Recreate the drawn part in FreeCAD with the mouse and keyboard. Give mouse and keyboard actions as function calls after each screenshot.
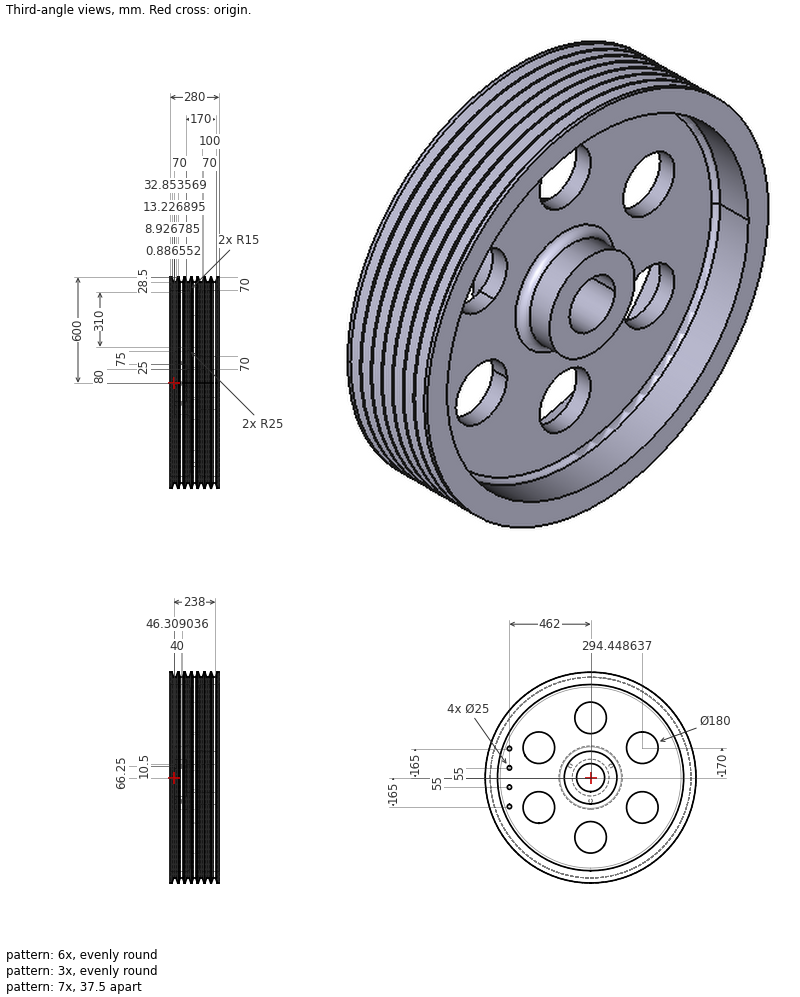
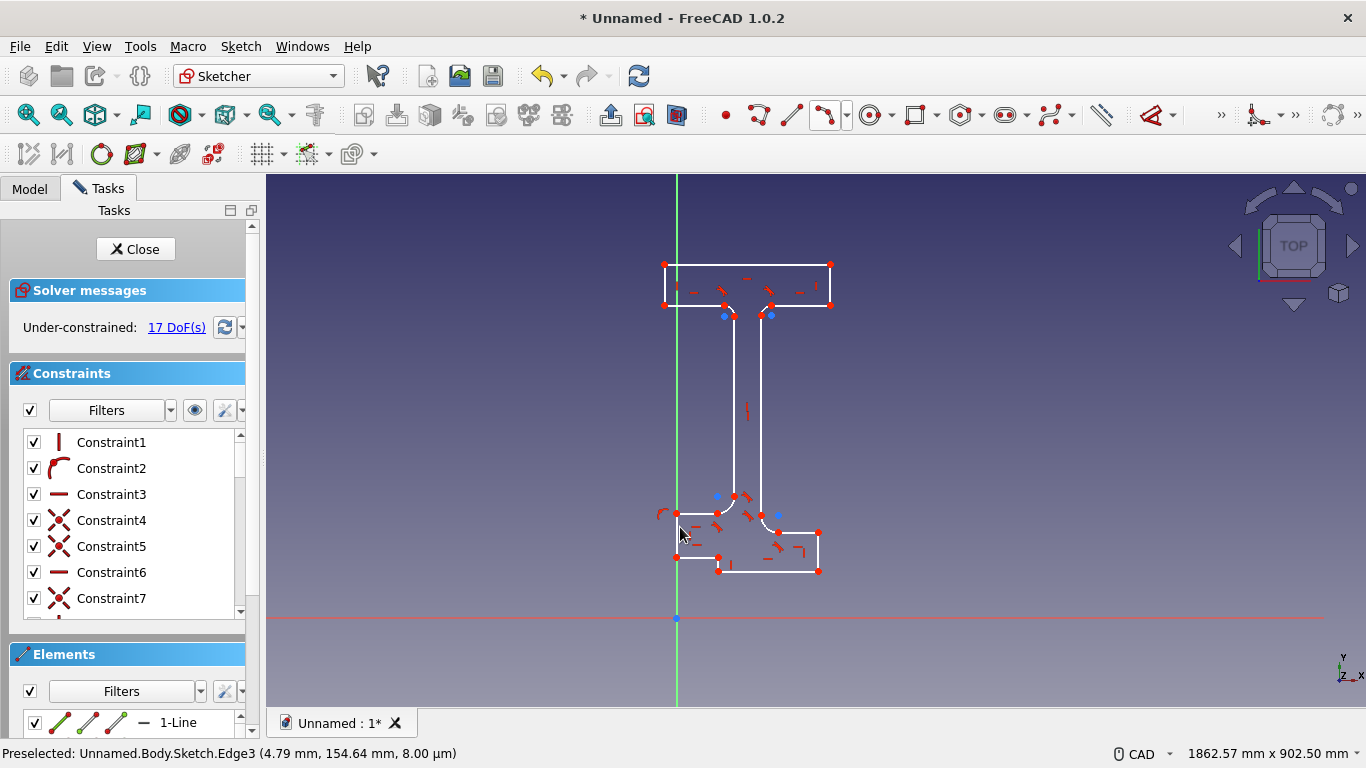
scroll(725, 512, up, 3)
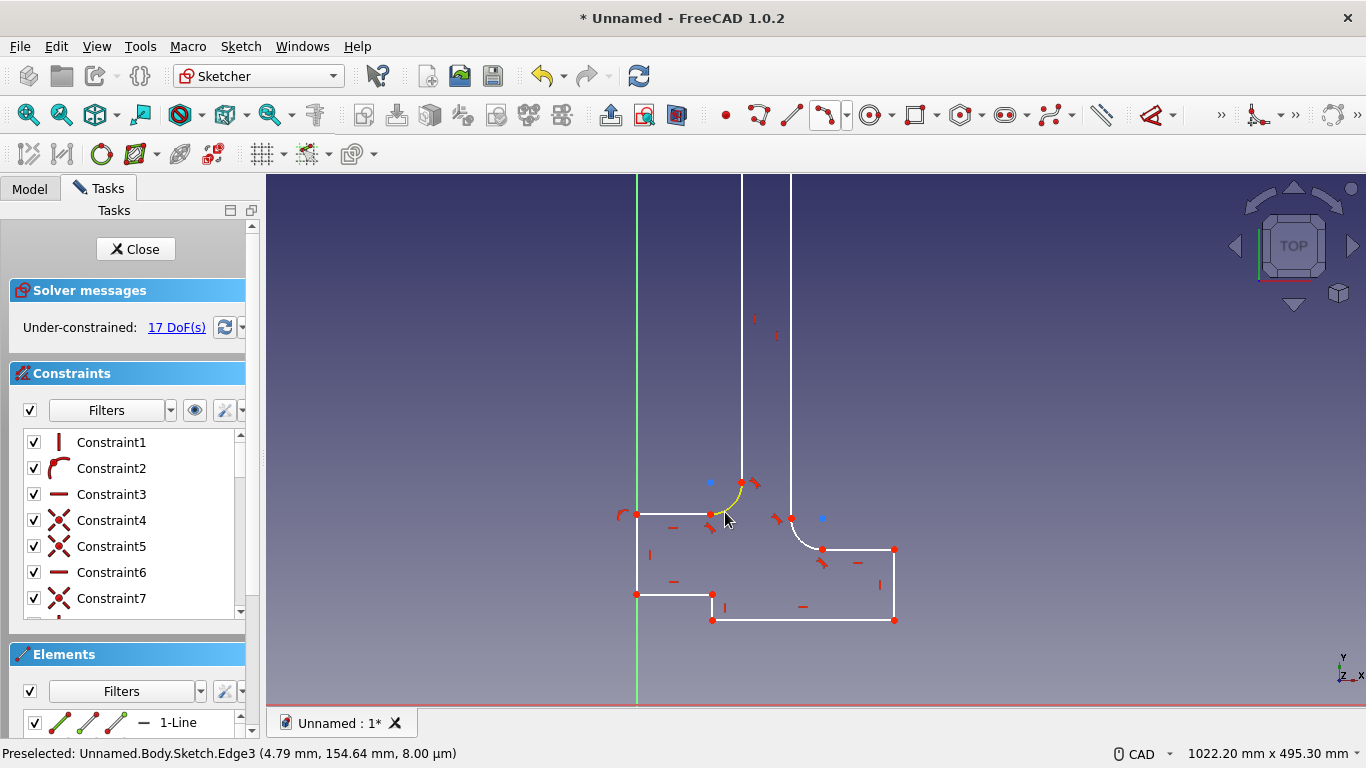
click(725, 511)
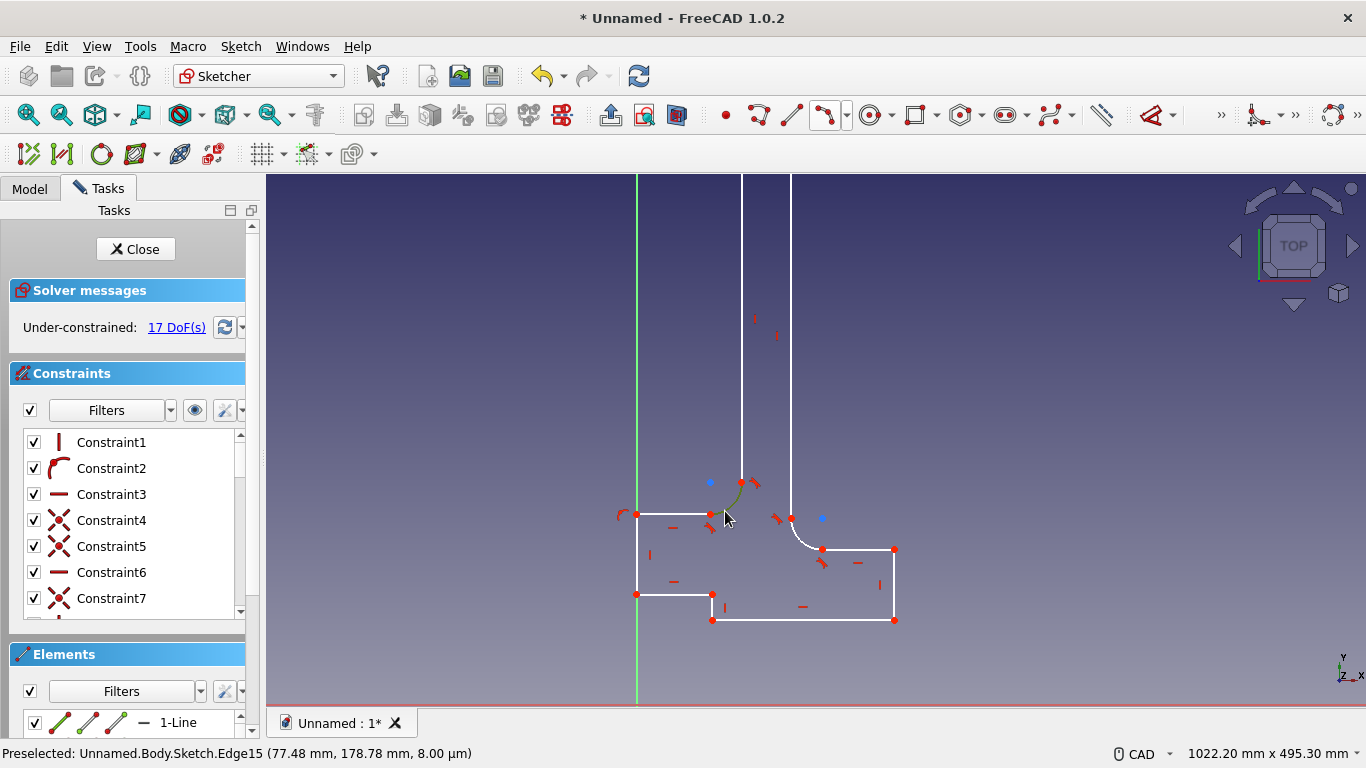
click(795, 532)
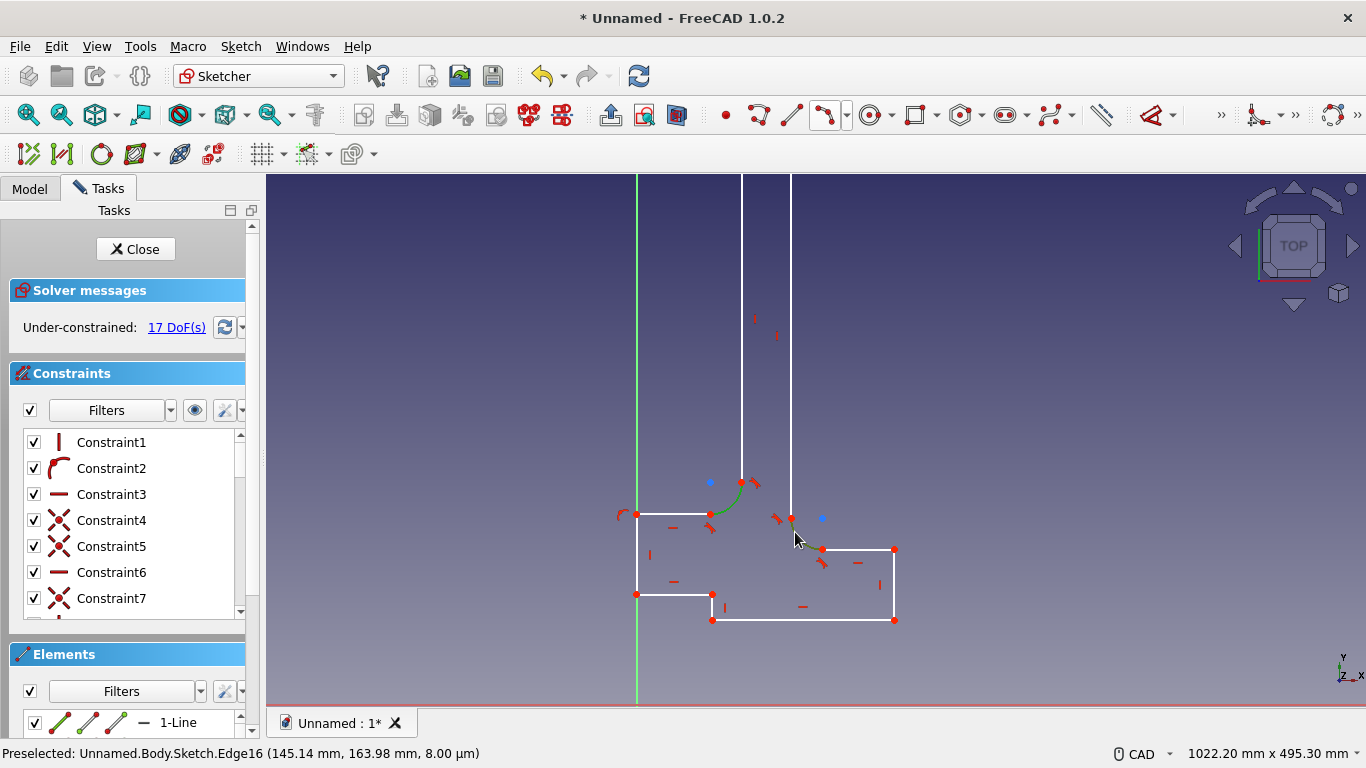
key(e)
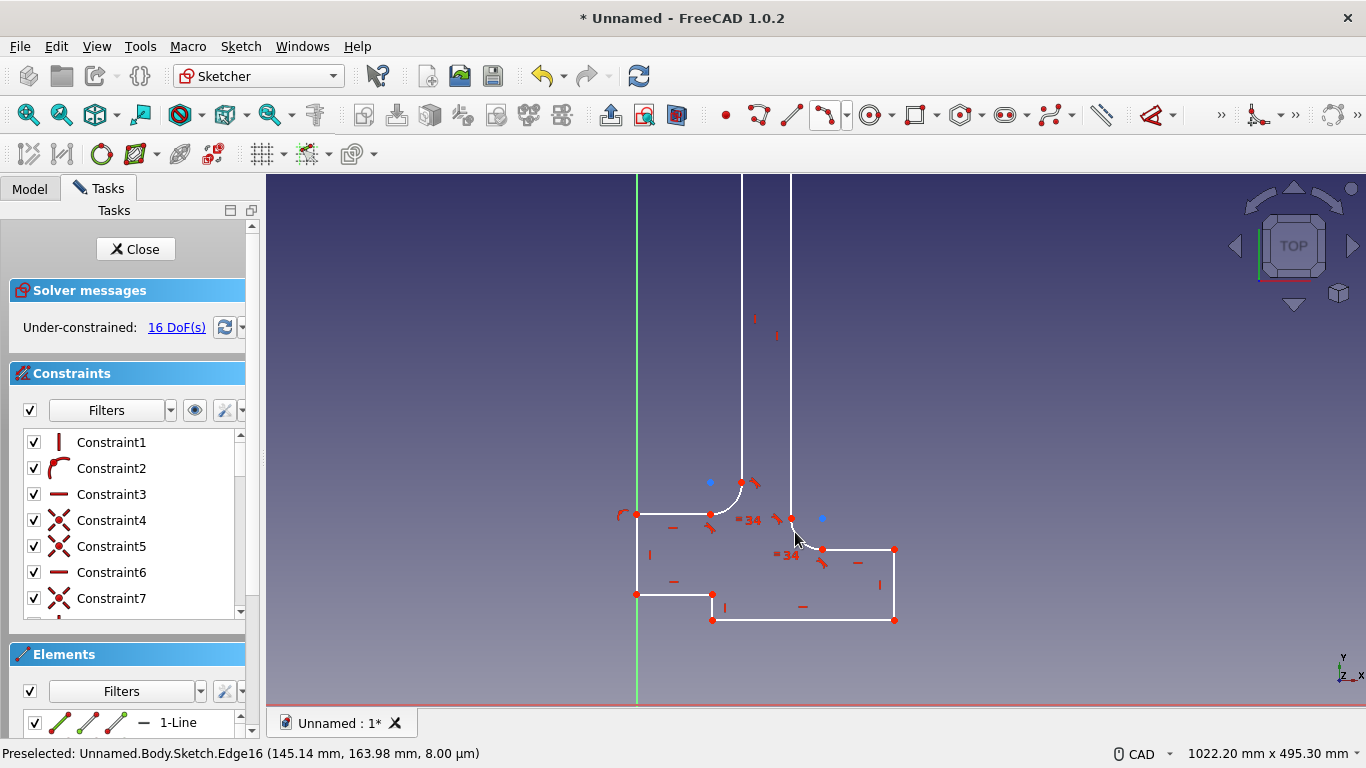
scroll(725, 511, down, 3)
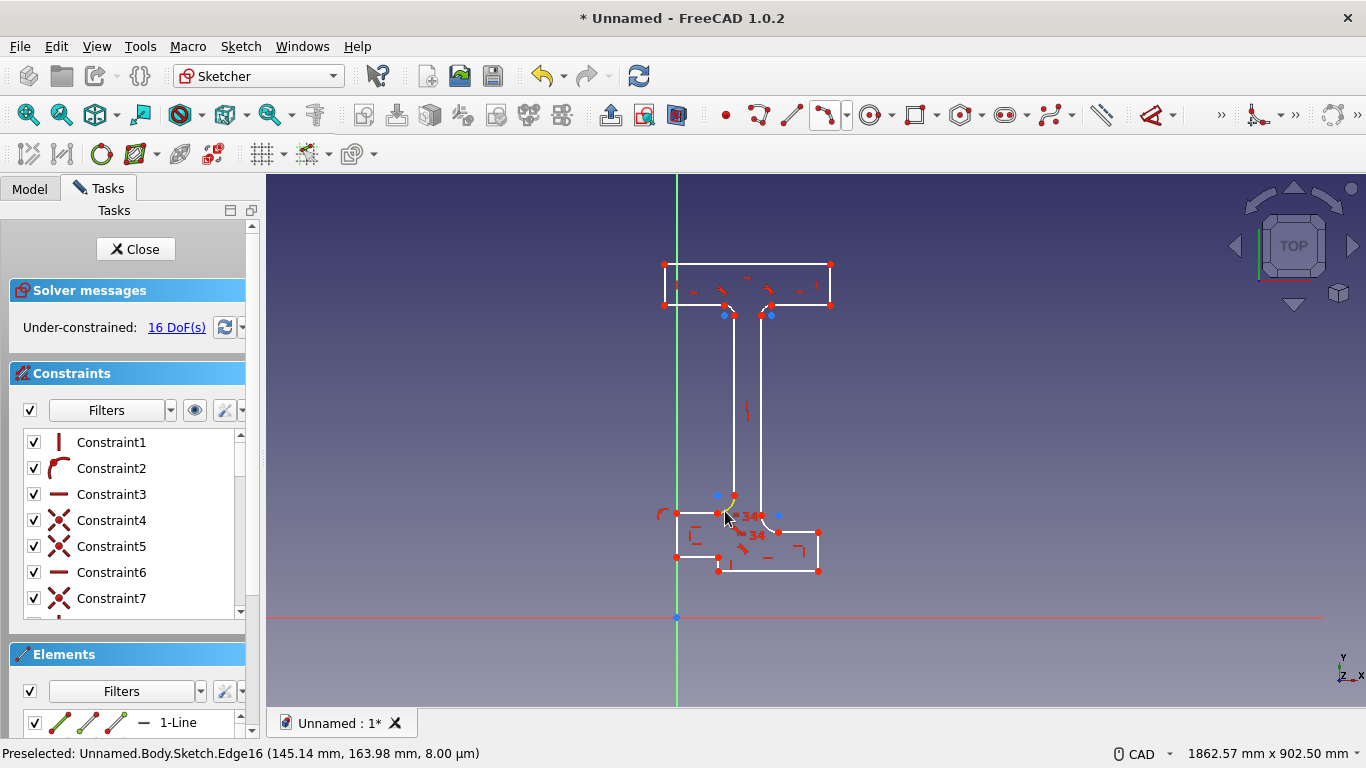
scroll(764, 308, up, 3)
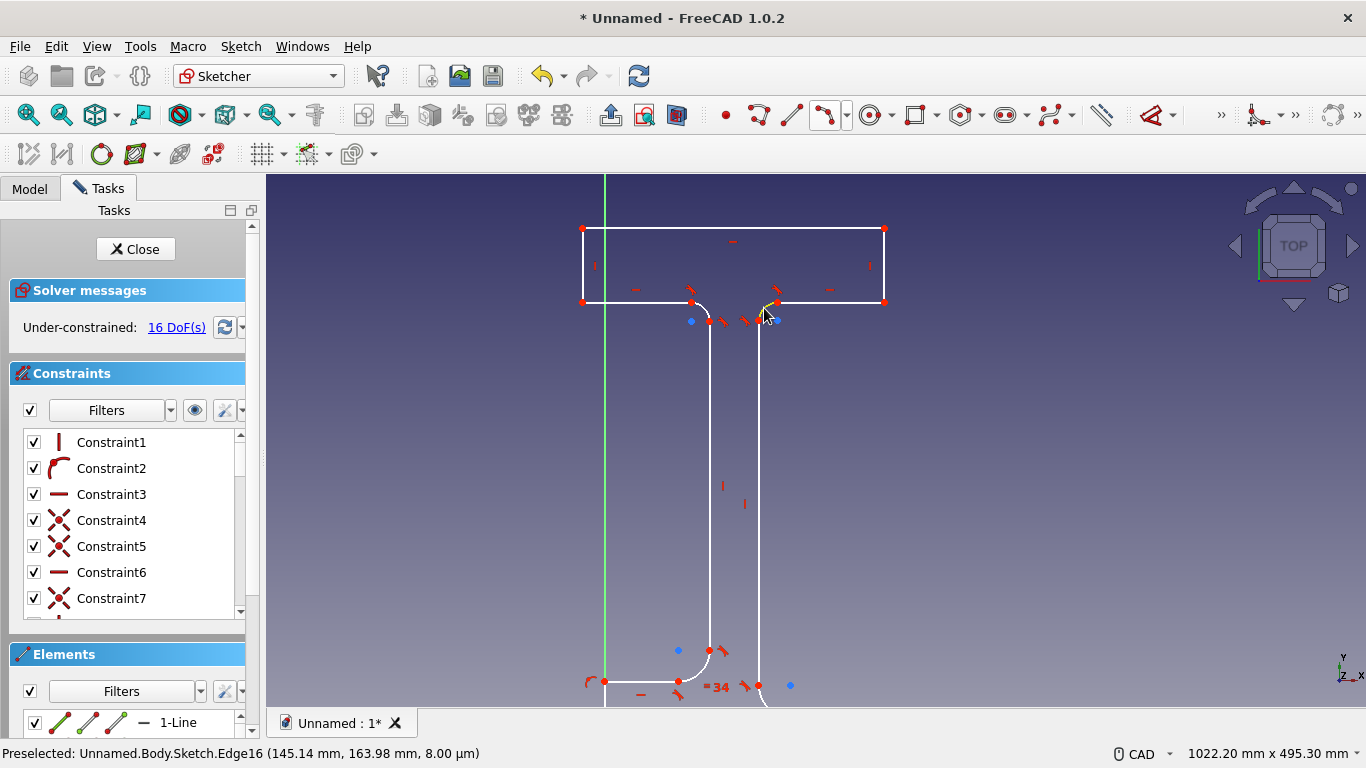
click(764, 308)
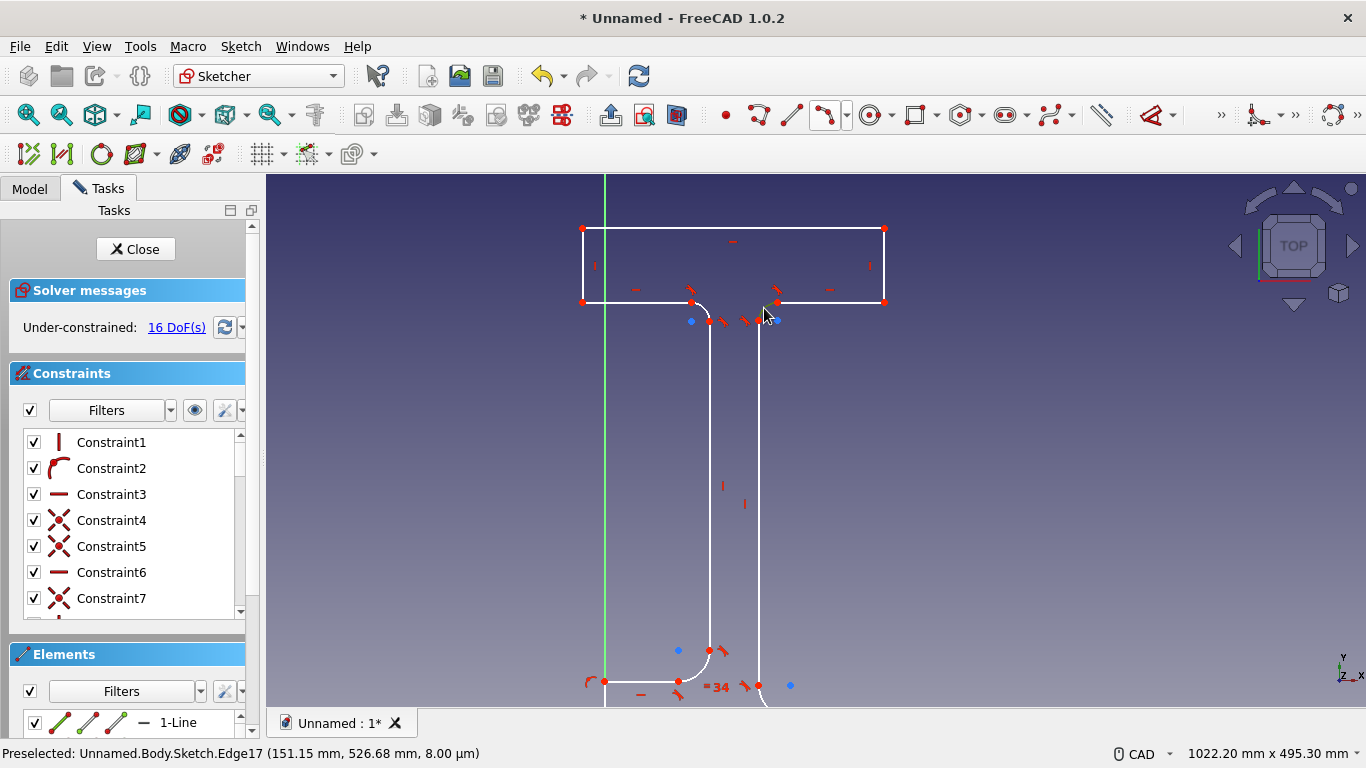
click(704, 308)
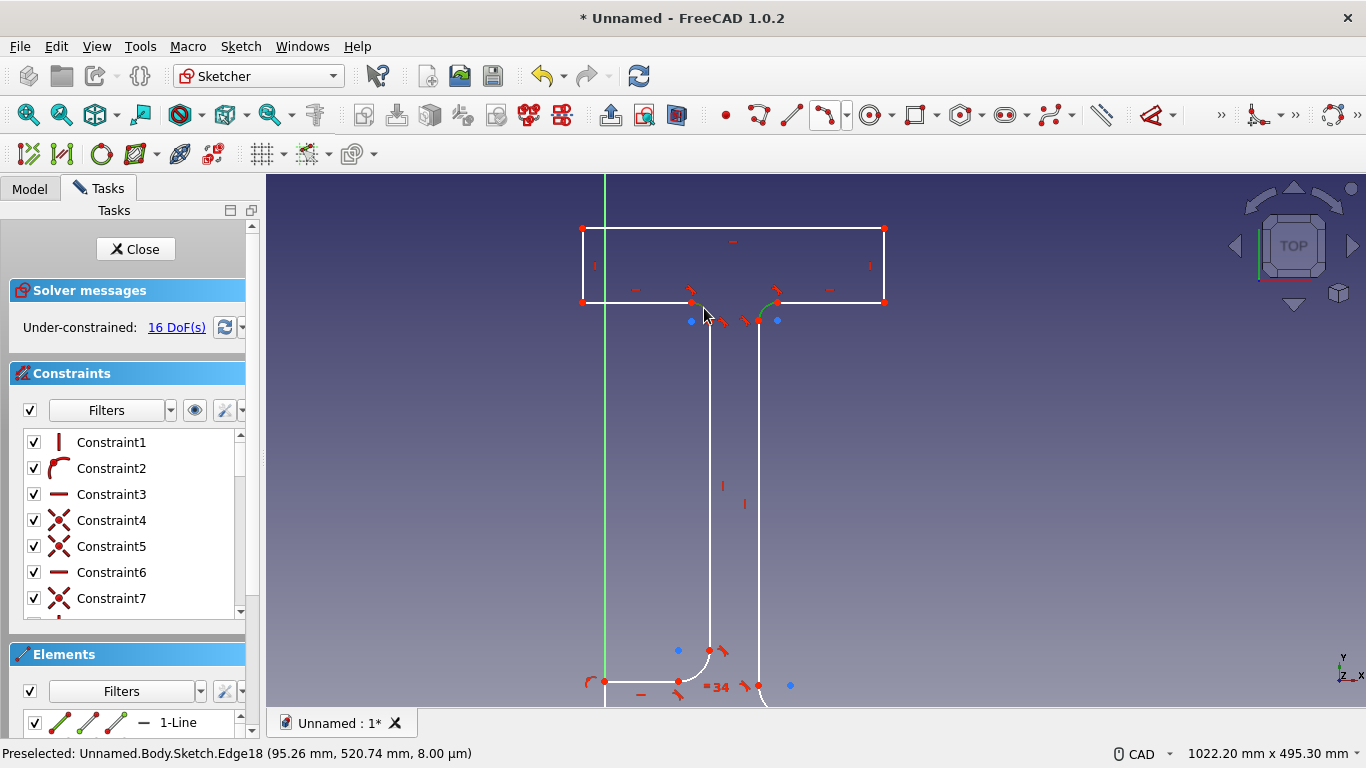
key(e)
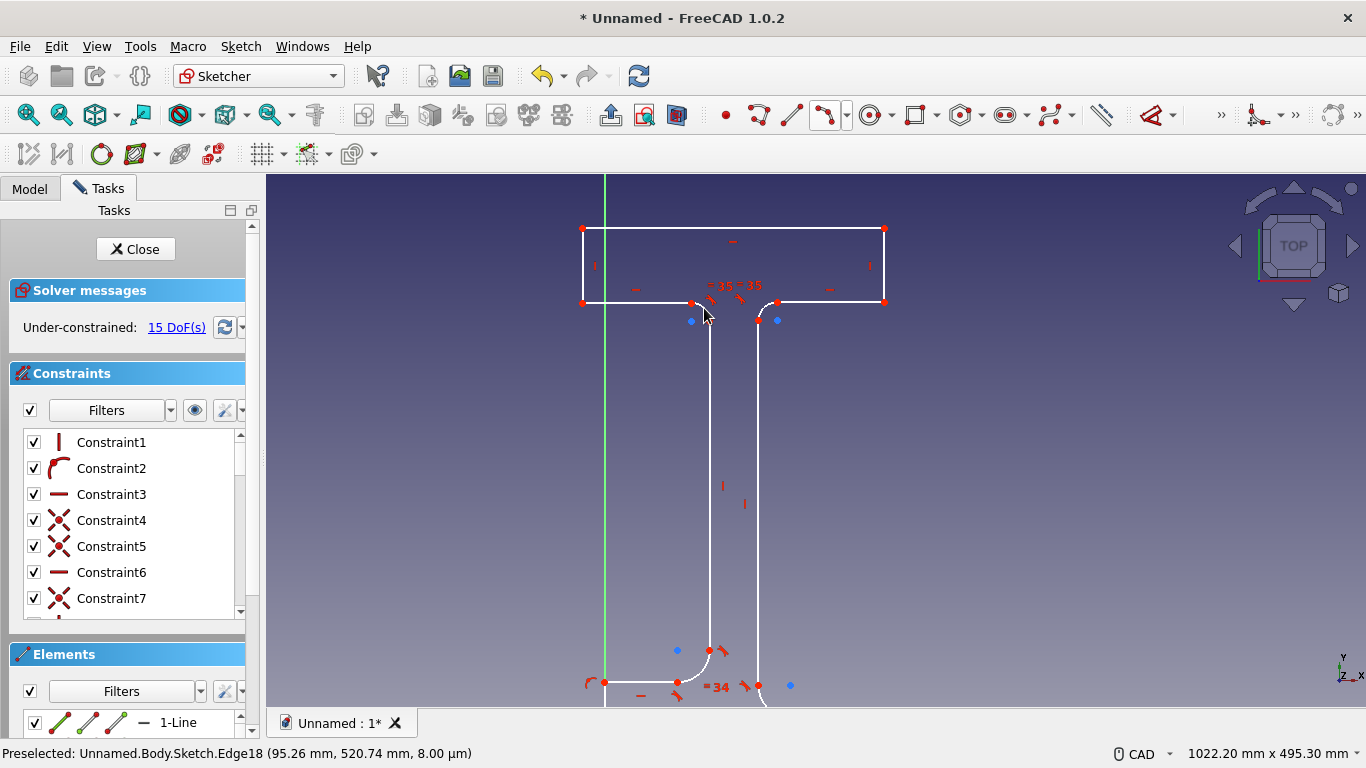
key(d)